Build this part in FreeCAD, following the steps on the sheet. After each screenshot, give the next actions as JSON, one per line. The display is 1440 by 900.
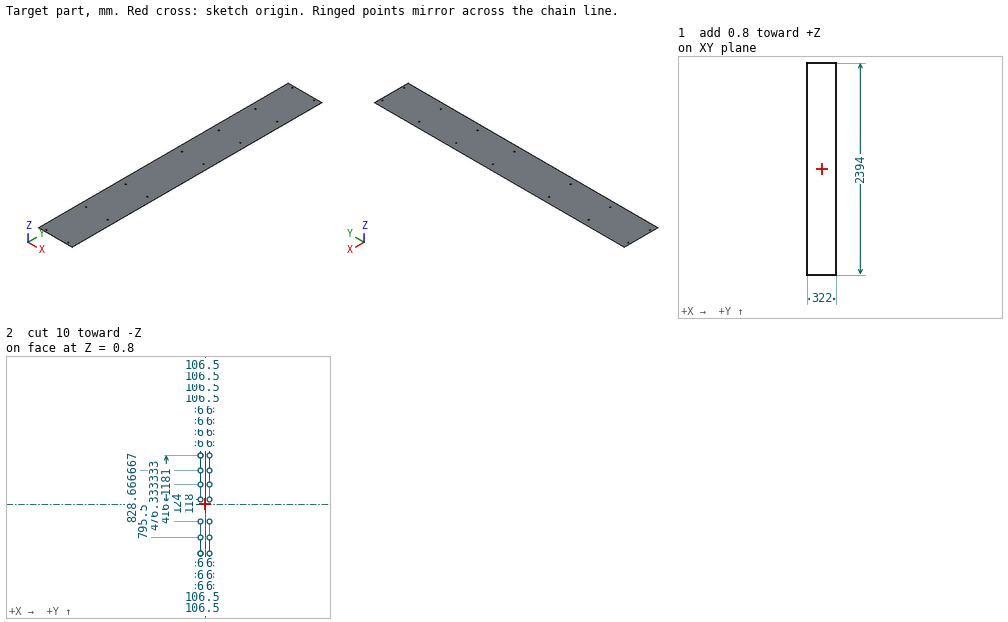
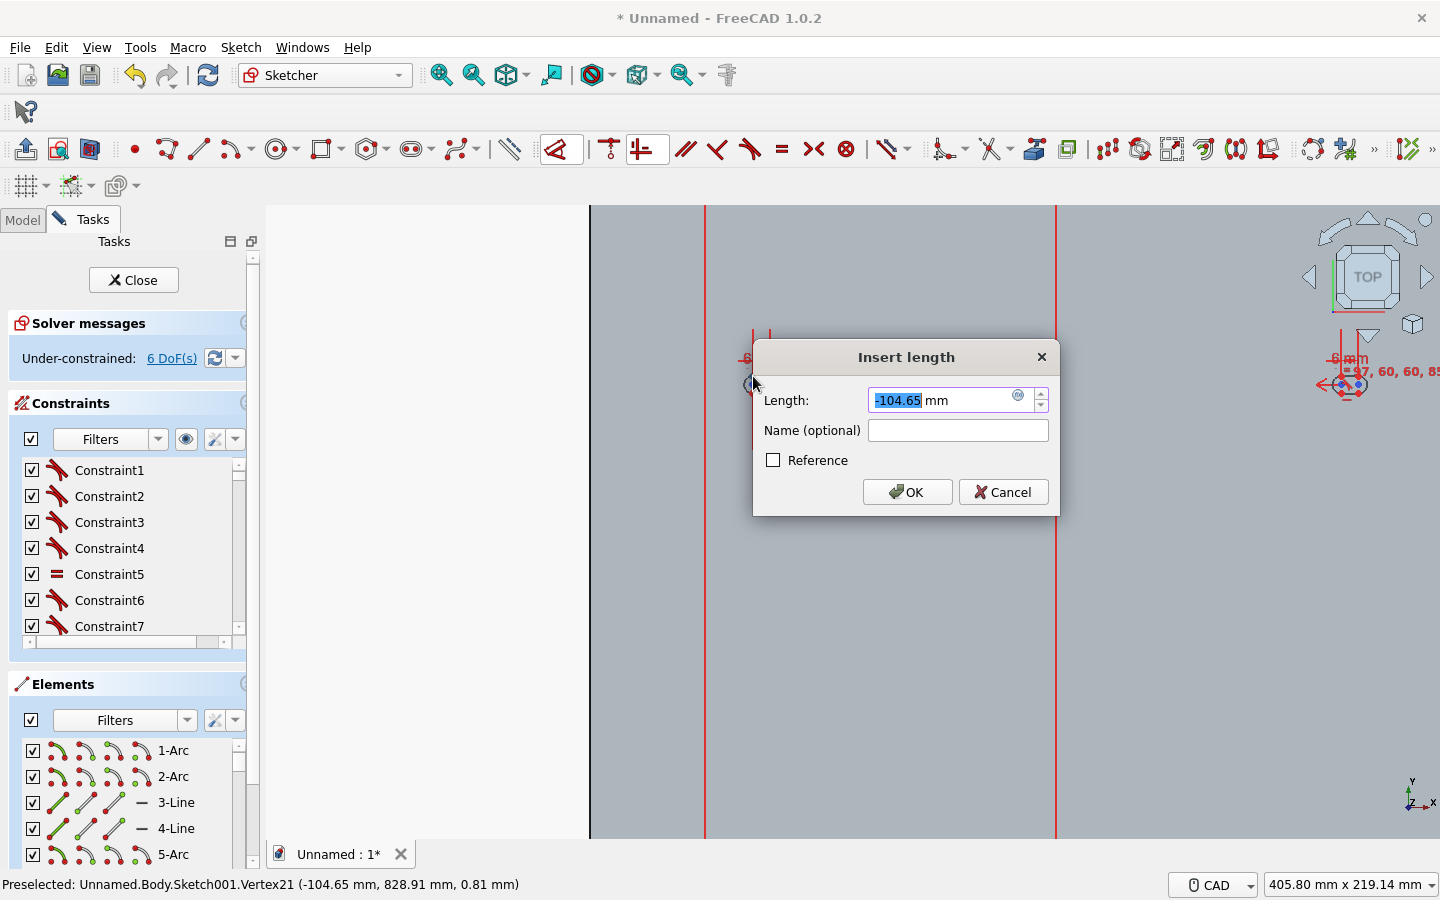
{"action": "type", "text": "-106.5"}
{"action": "key", "text": "Return"}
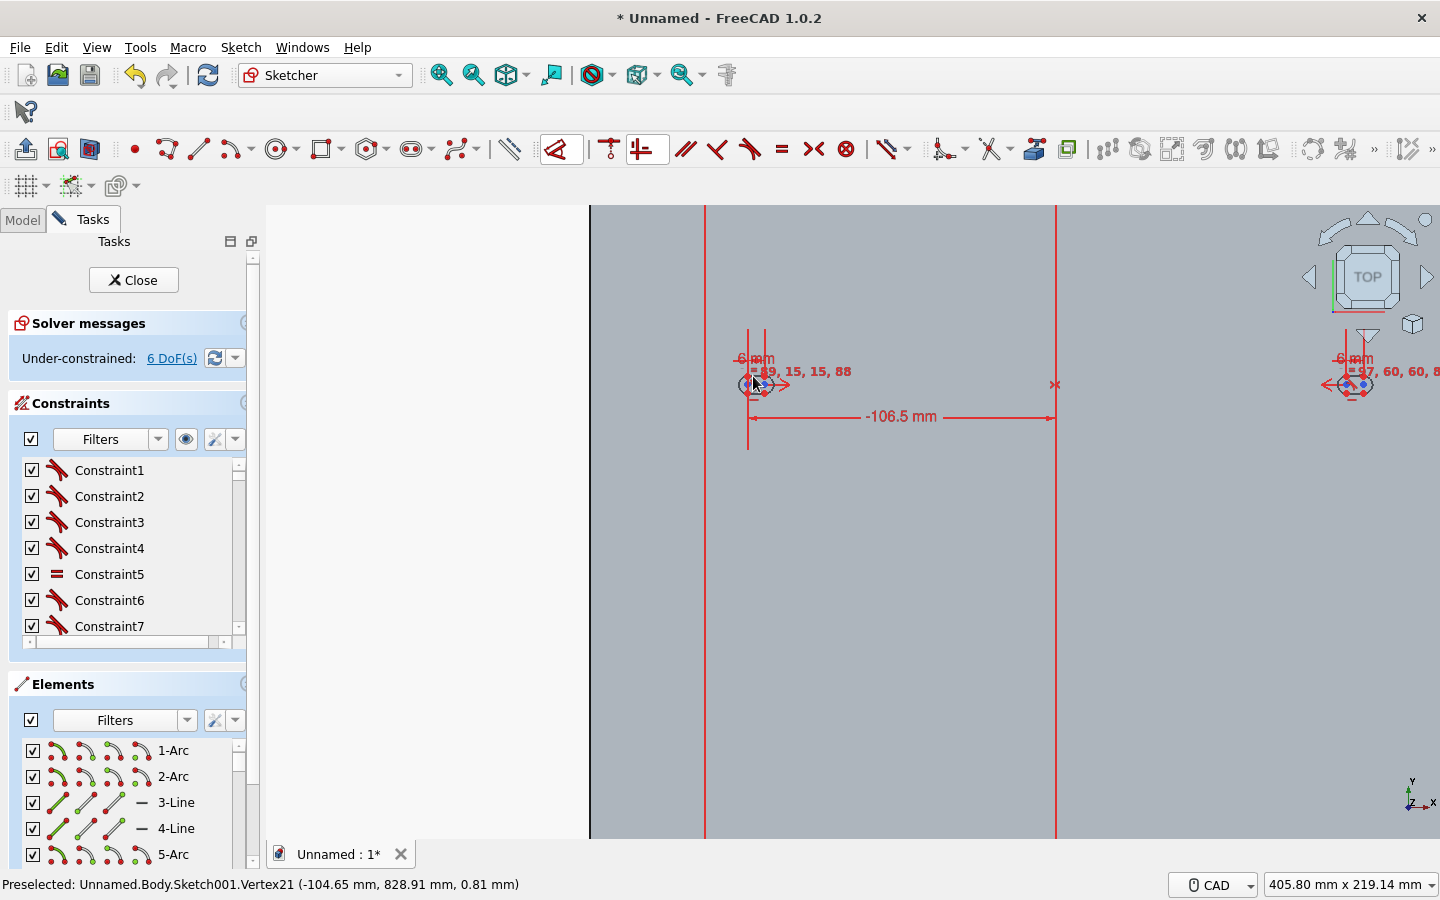
{"action": "scroll", "coordinate": [767, 376], "scroll_direction": "down", "scroll_amount": 14}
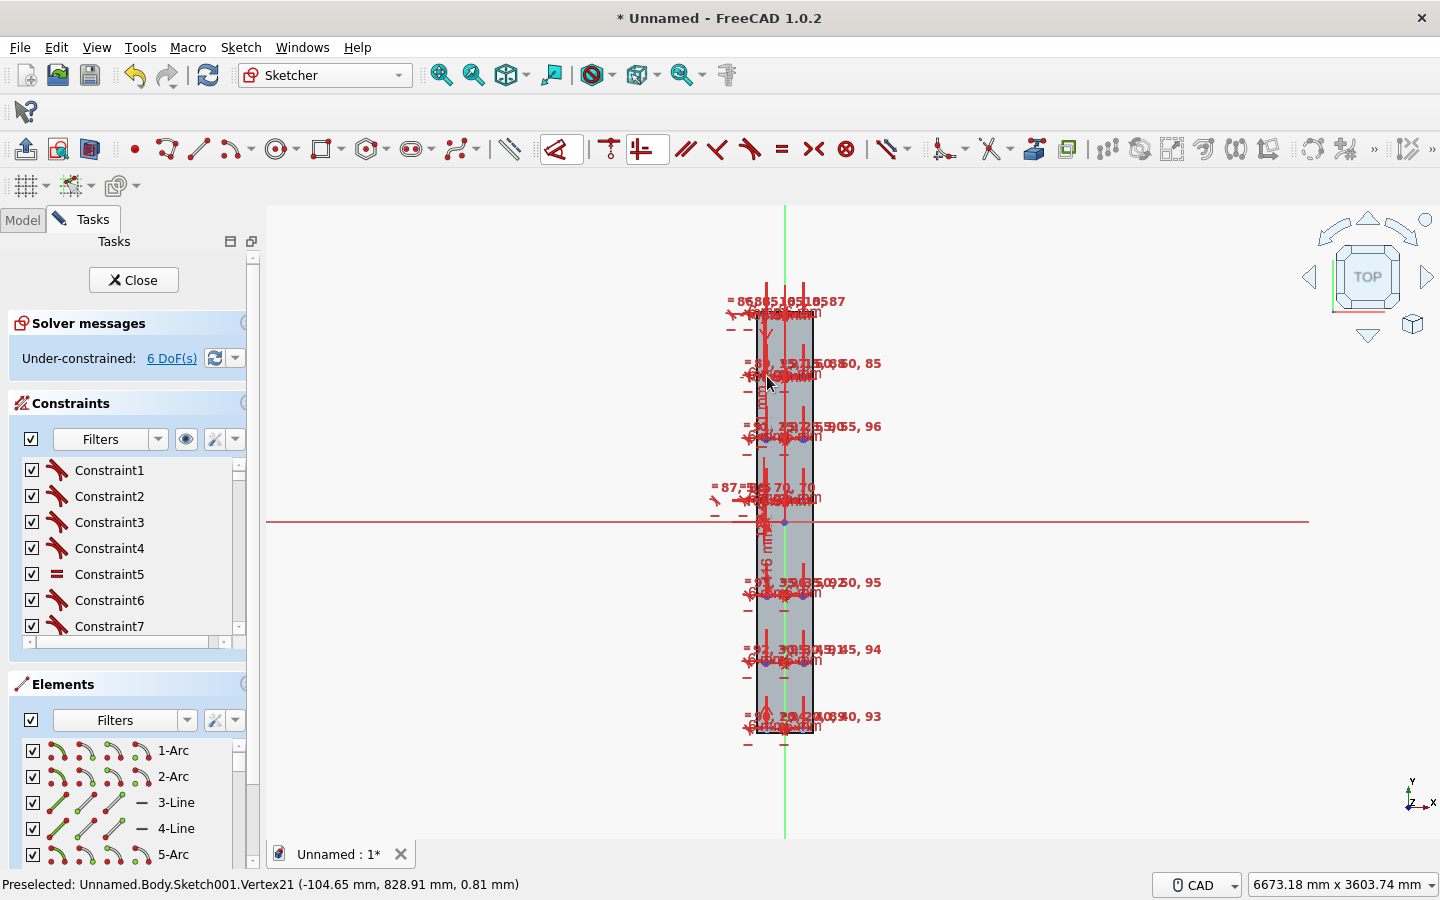
{"action": "scroll", "coordinate": [766, 439], "scroll_direction": "up", "scroll_amount": 14}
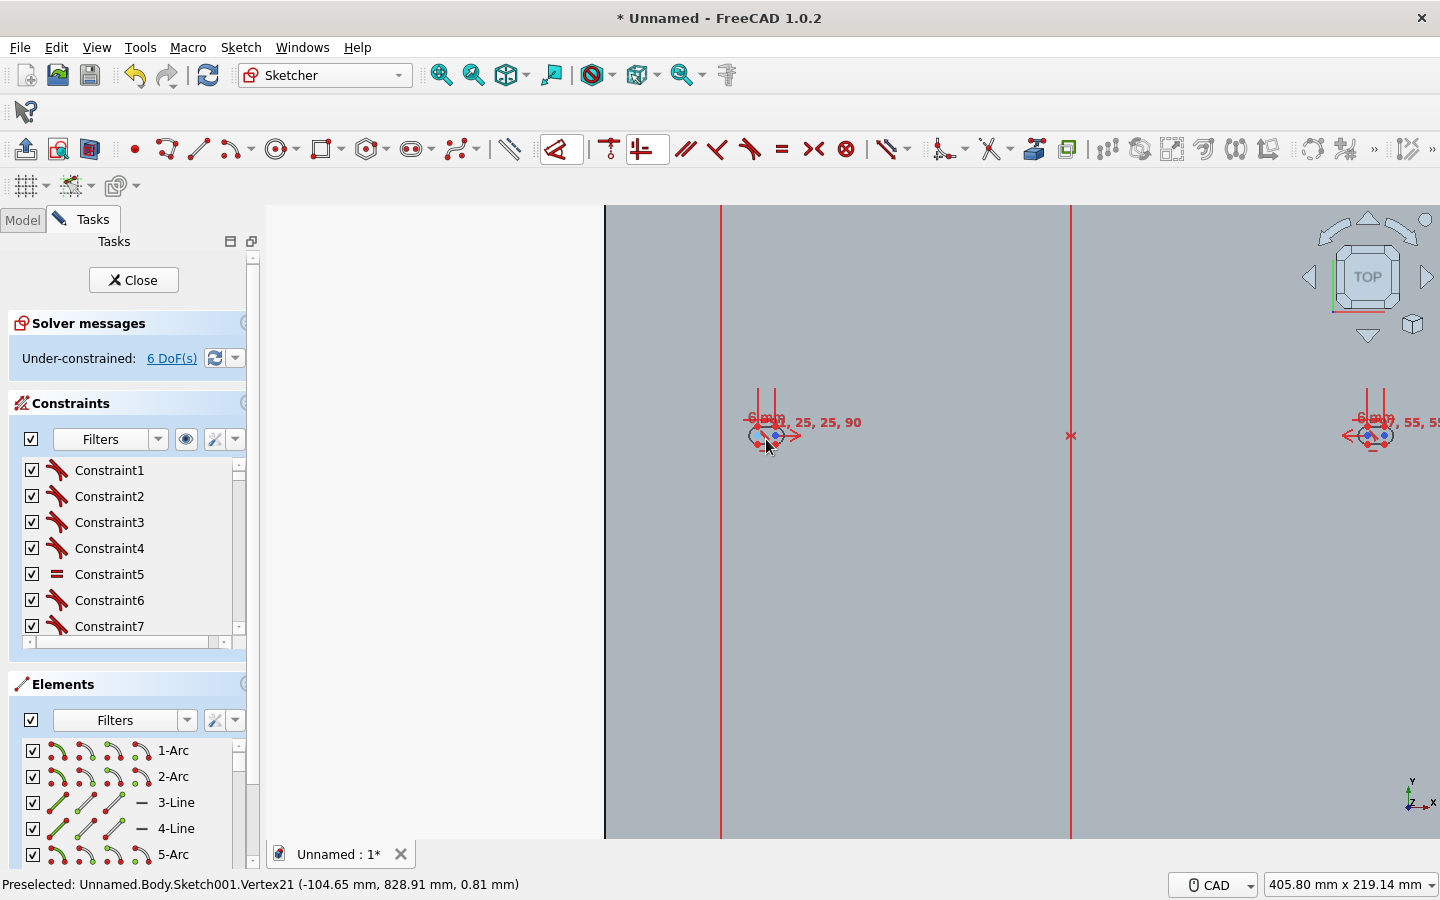
{"action": "left_click", "coordinate": [758, 427]}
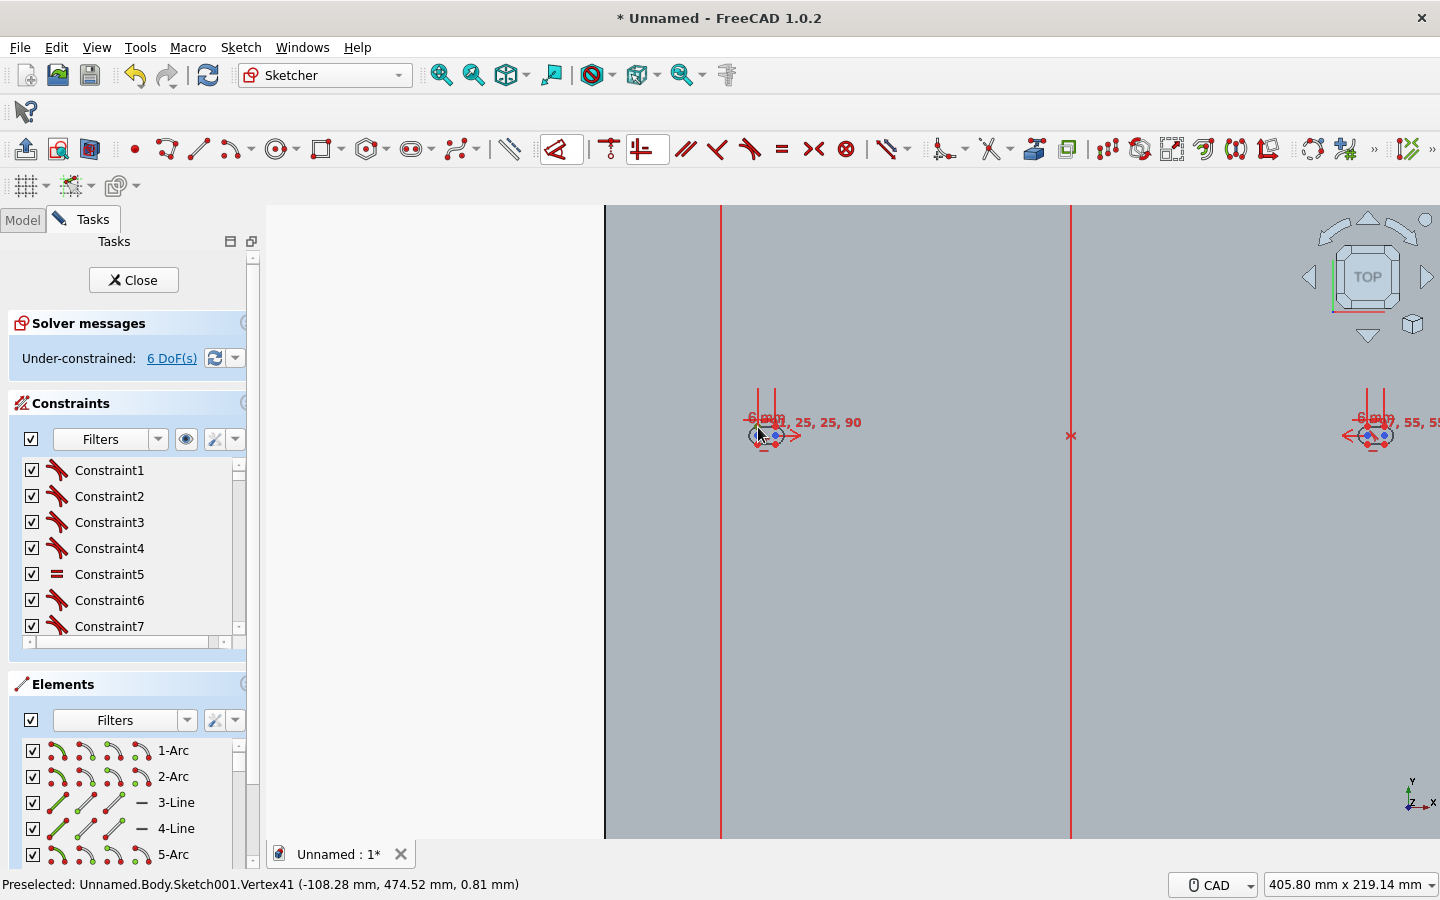
{"action": "key", "text": "l"}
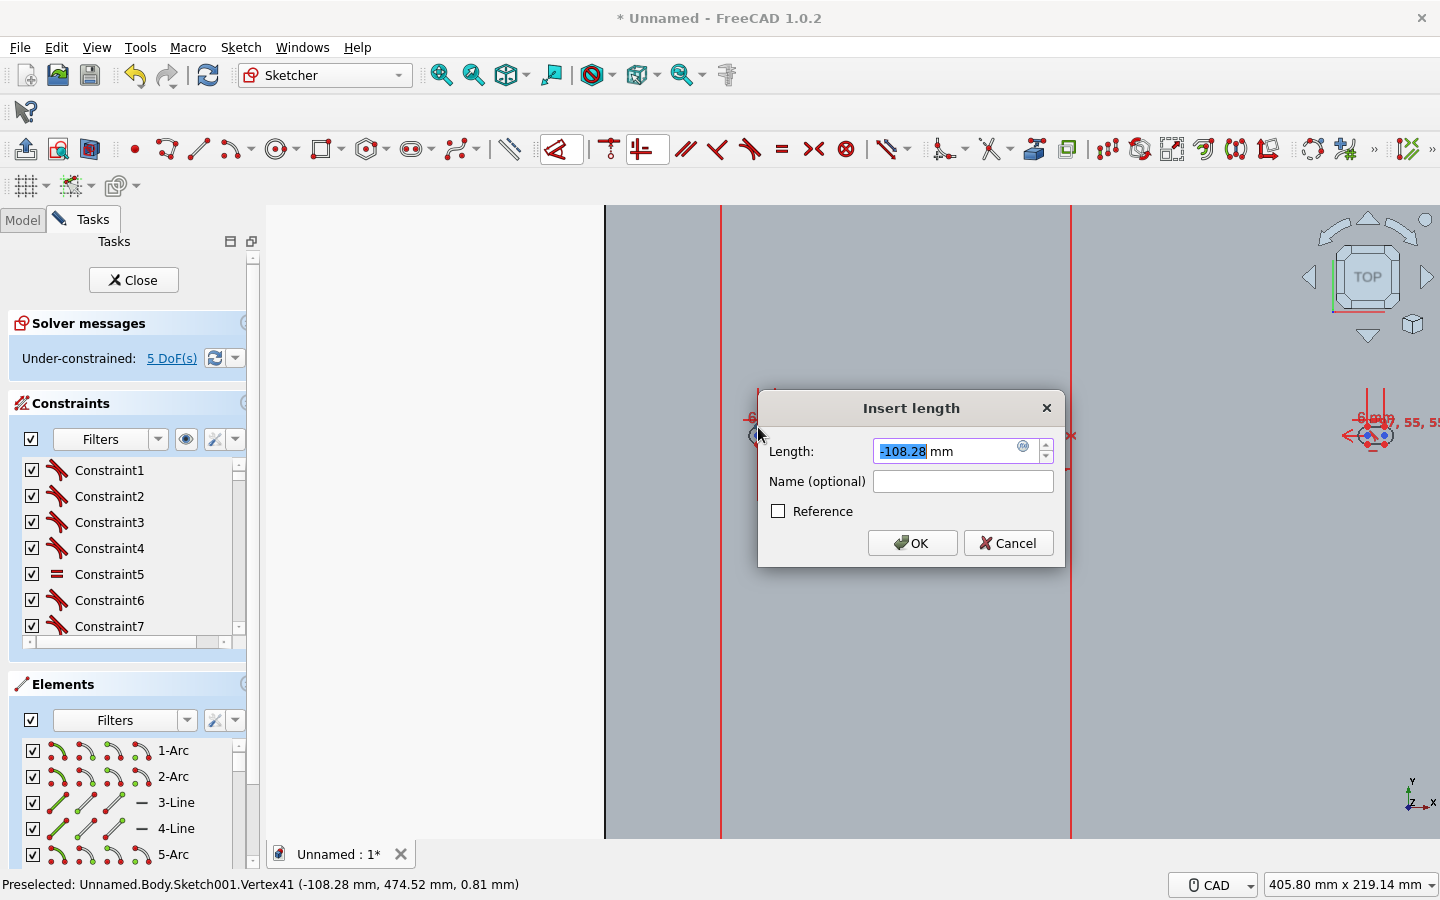
{"action": "type", "text": "-106.5"}
{"action": "key", "text": "Return"}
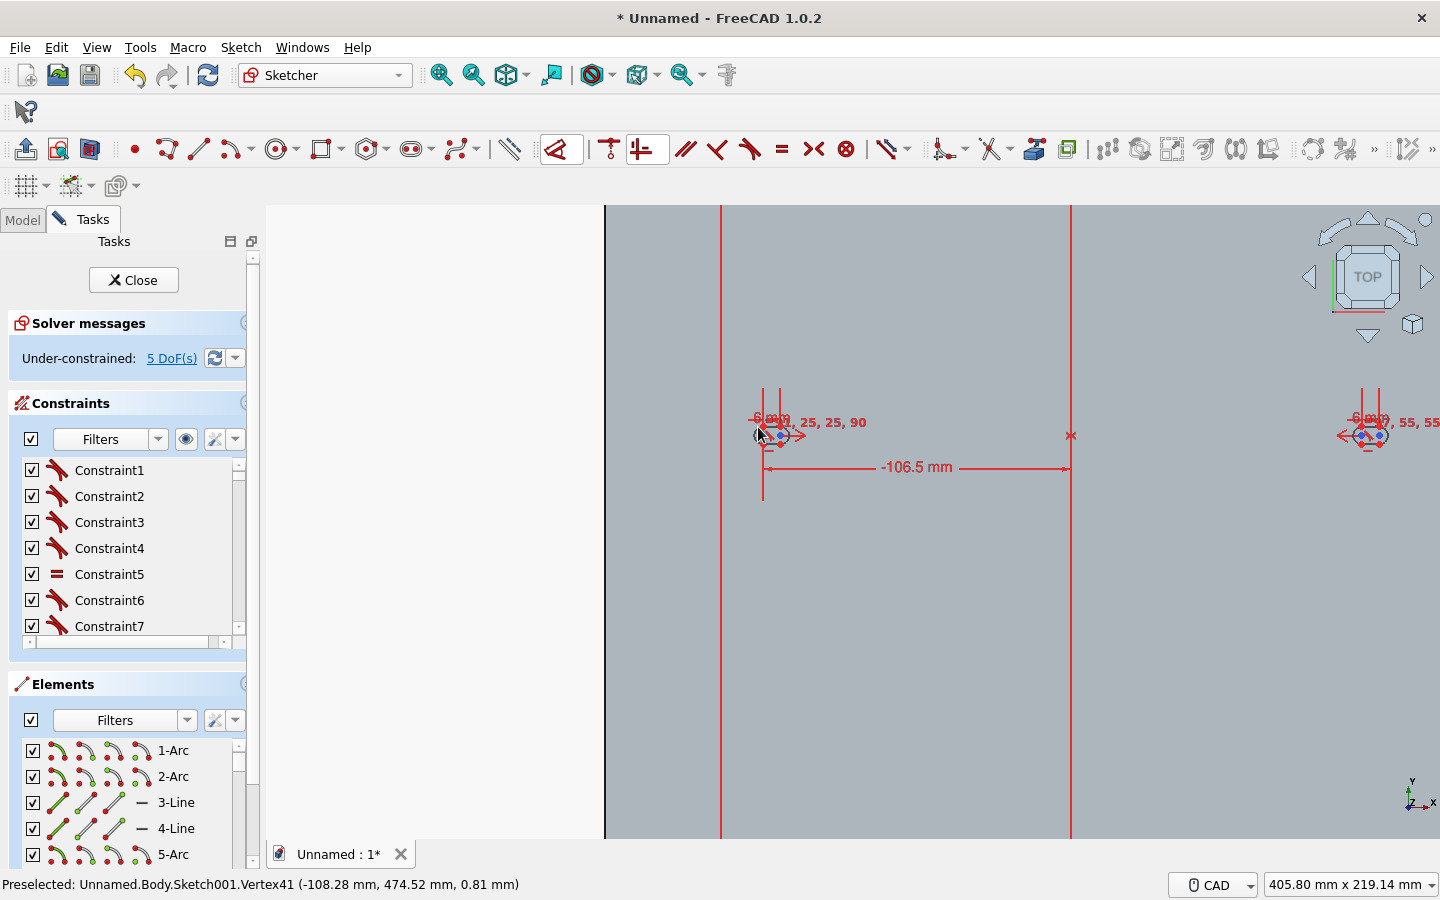
{"action": "scroll", "coordinate": [766, 439], "scroll_direction": "down", "scroll_amount": 14}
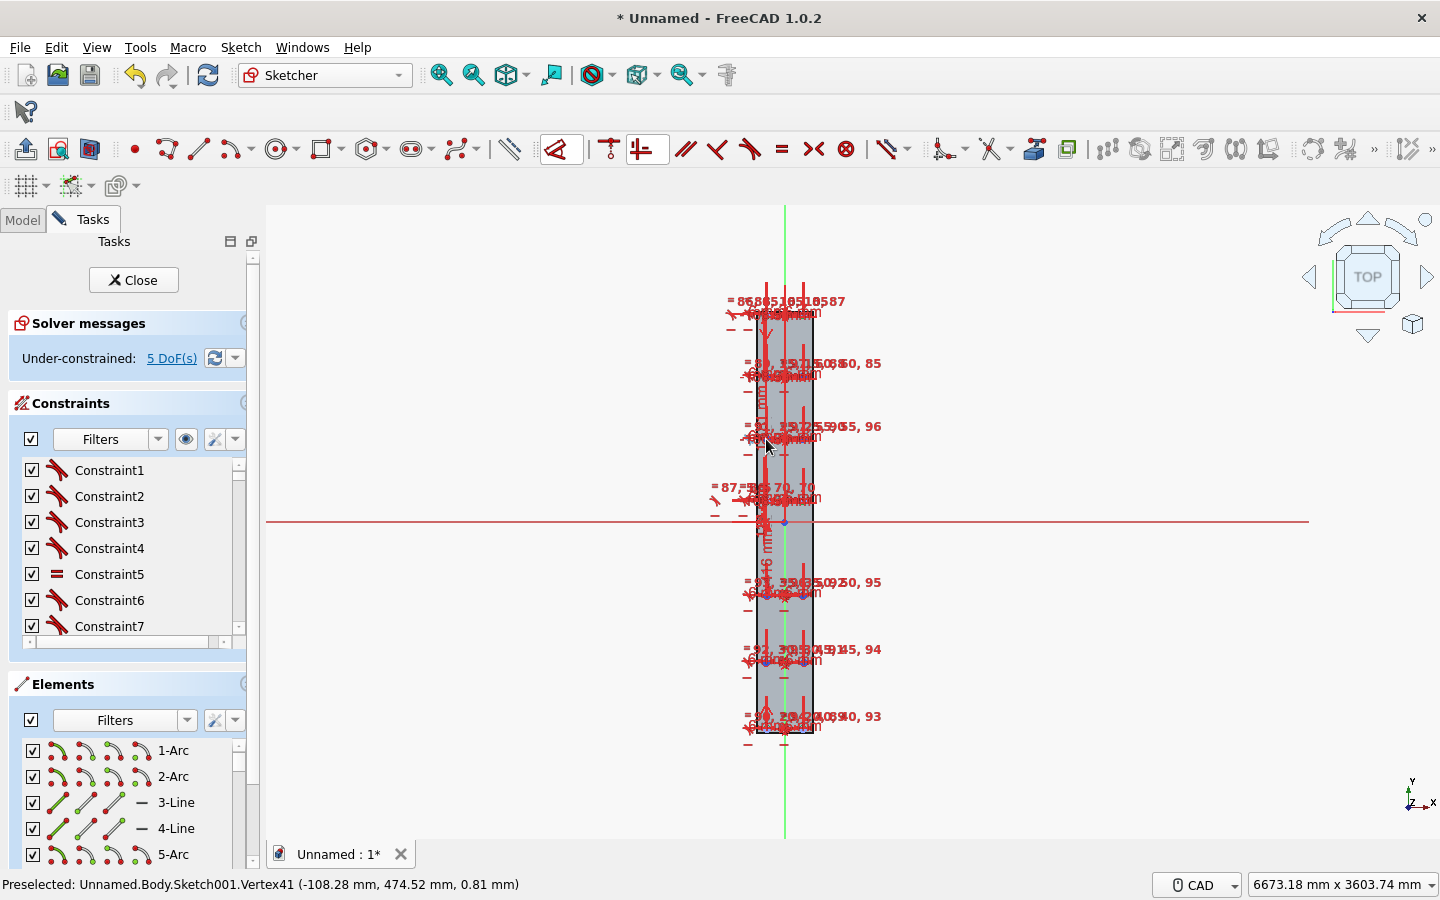
{"action": "scroll", "coordinate": [766, 662], "scroll_direction": "up", "scroll_amount": 14}